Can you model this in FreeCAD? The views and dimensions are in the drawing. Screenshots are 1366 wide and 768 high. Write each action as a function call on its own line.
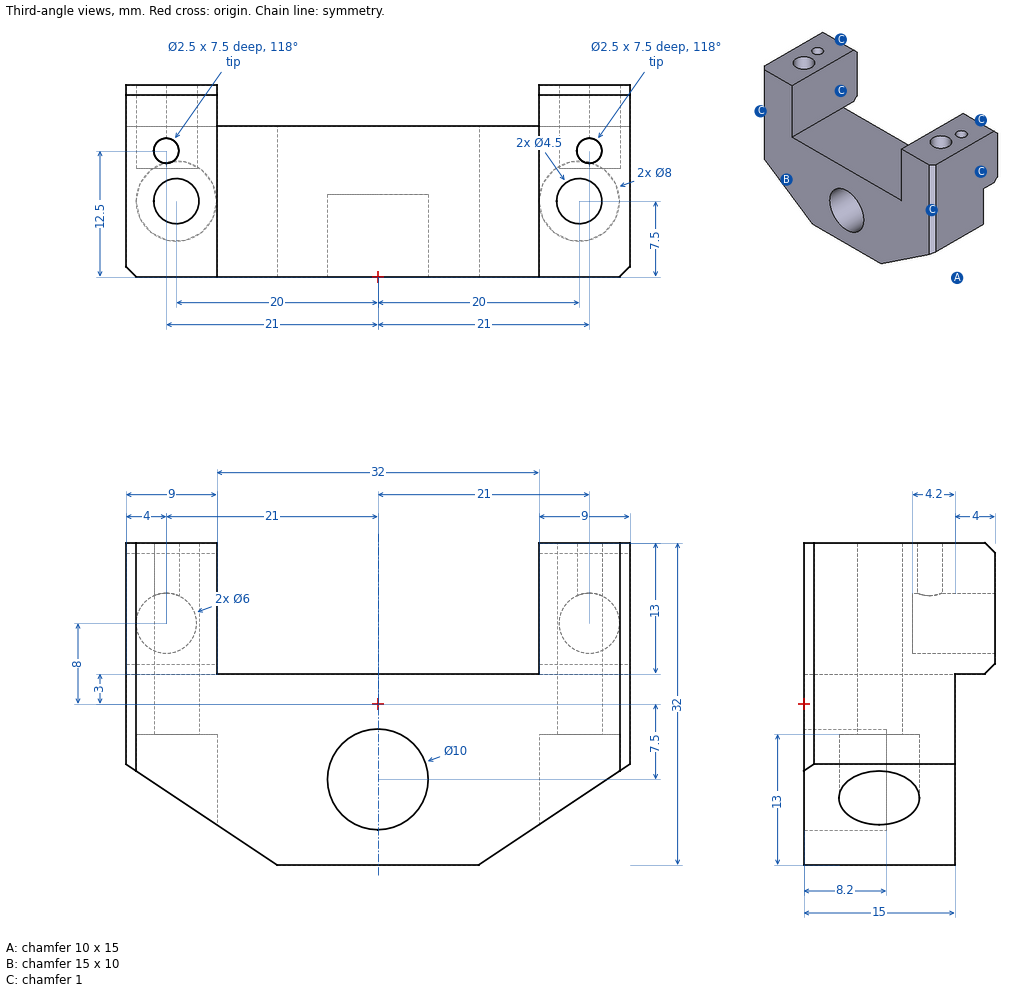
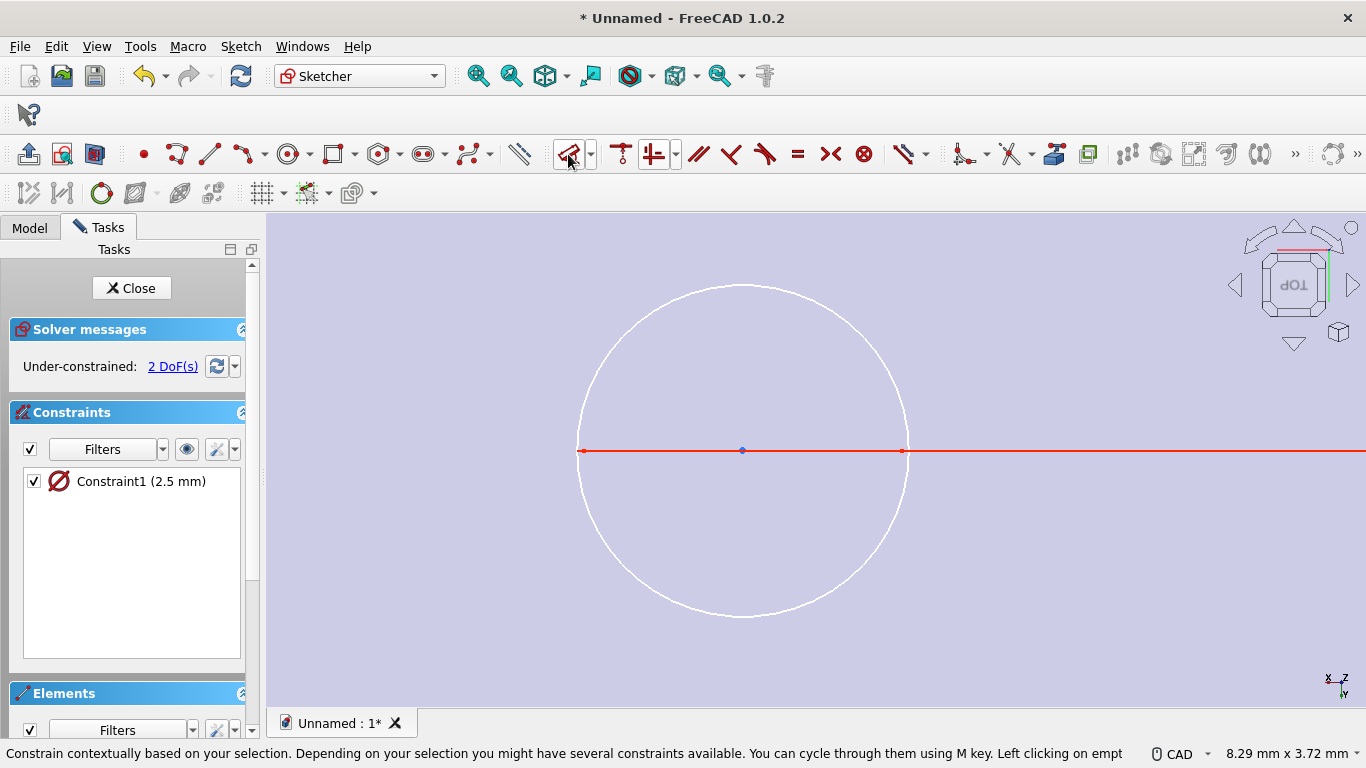
click(743, 451)
click(972, 485)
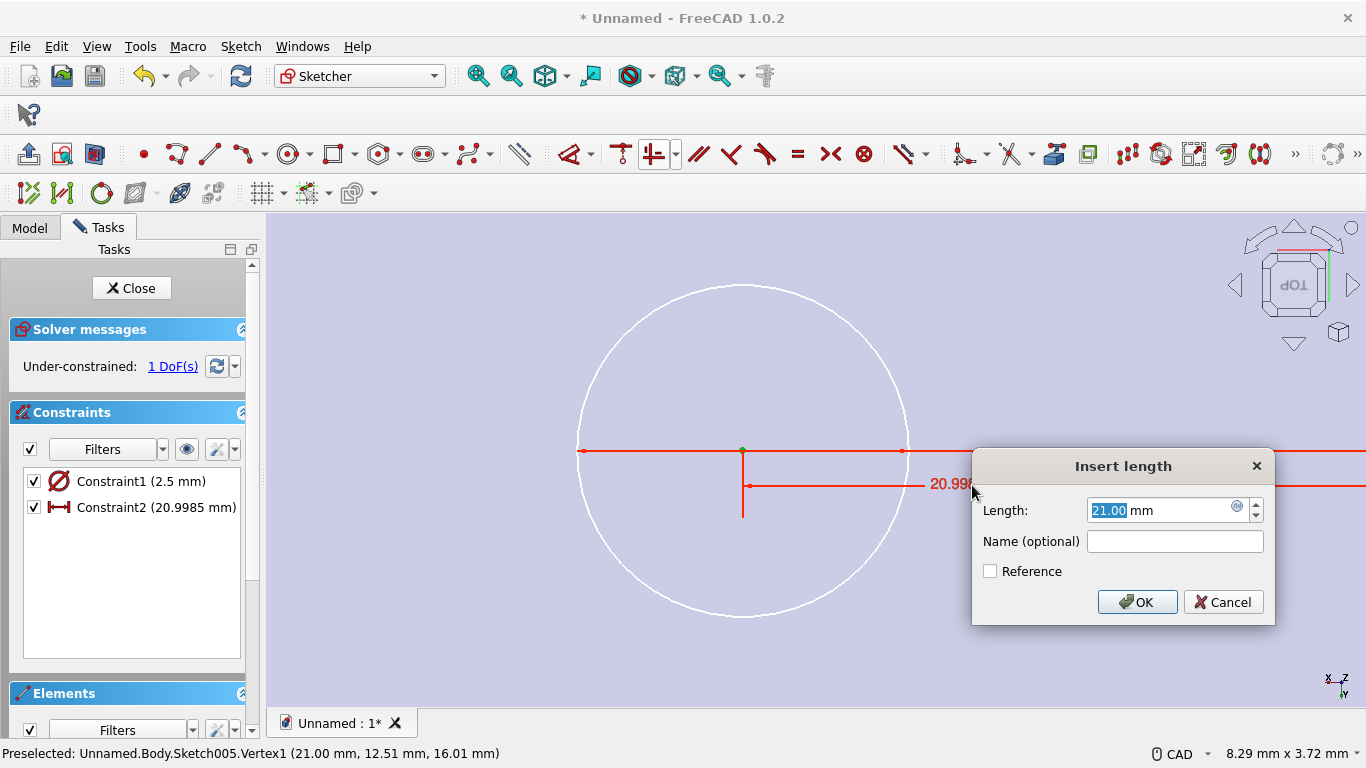
text(21)
key(Return)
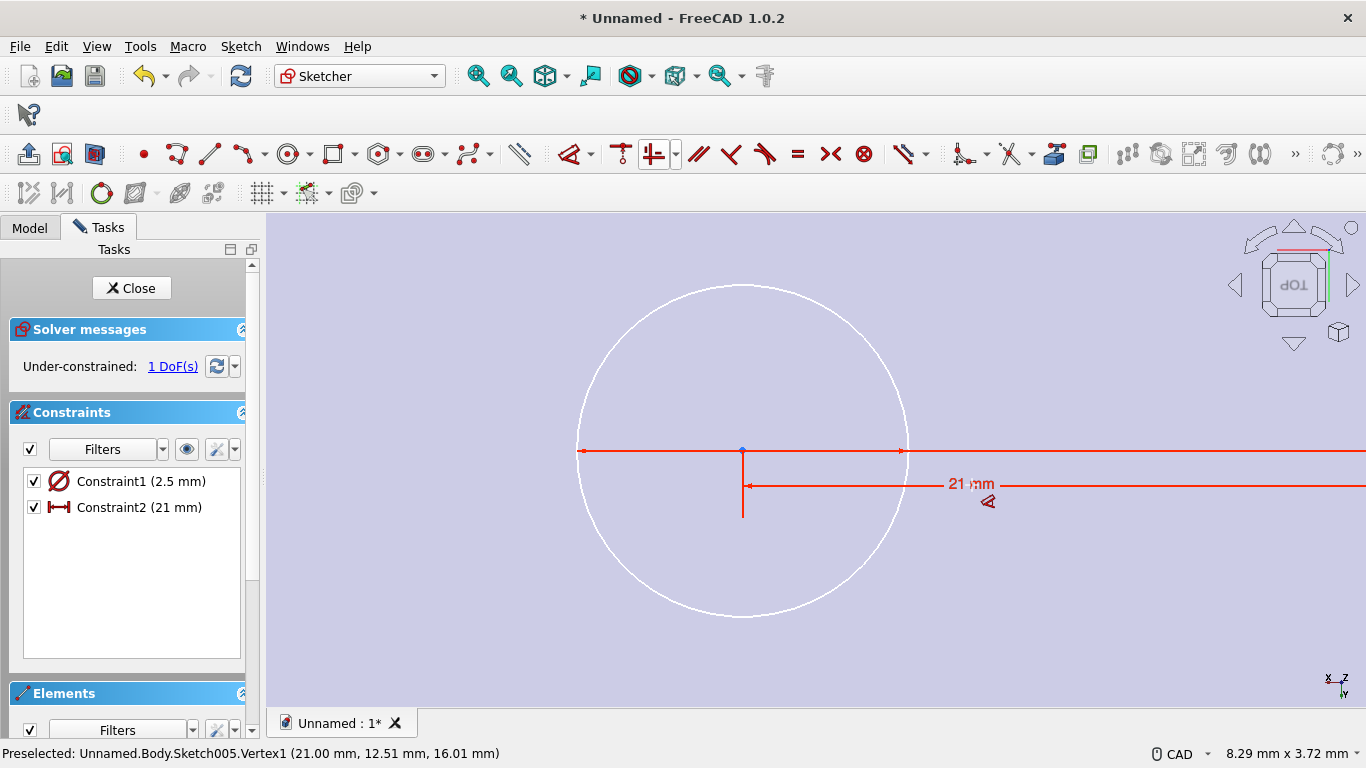
click(743, 451)
click(709, 346)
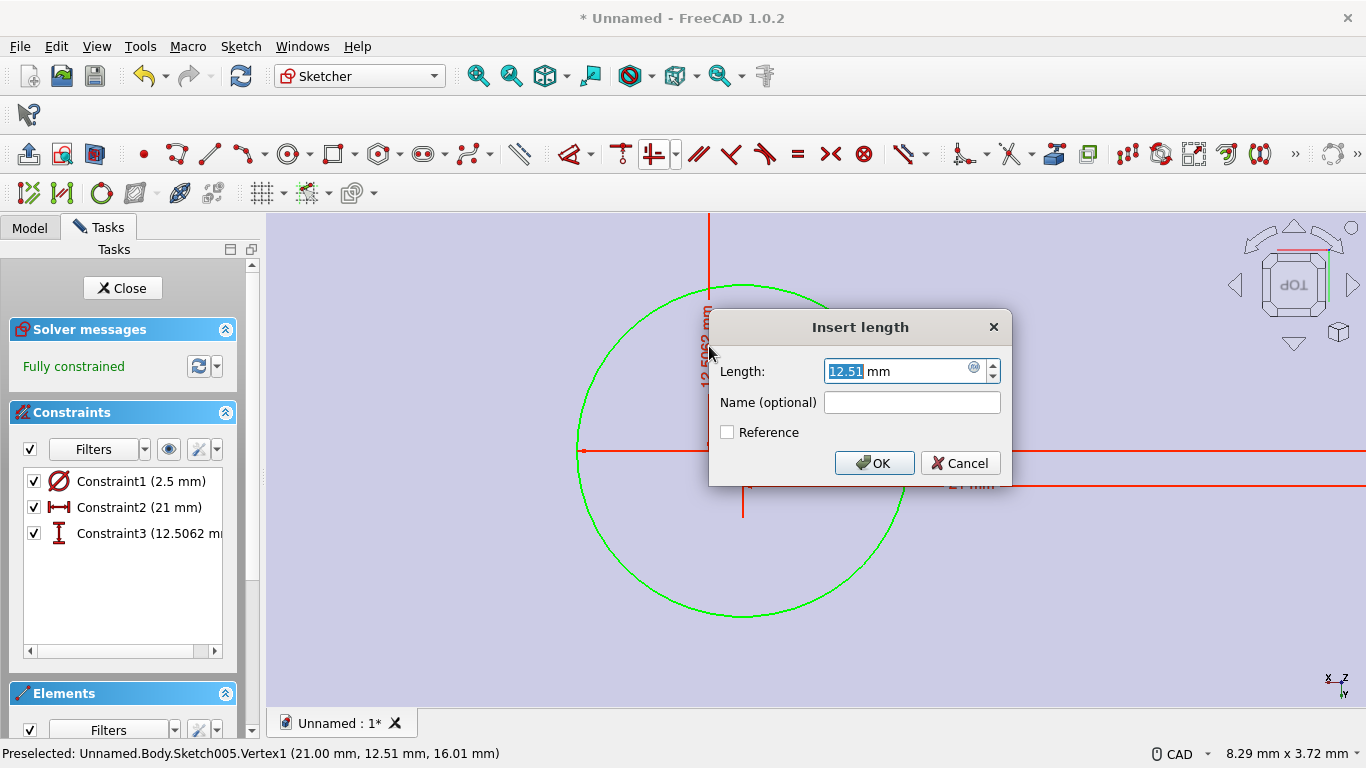
text(12.5)
key(Return)
key(Escape)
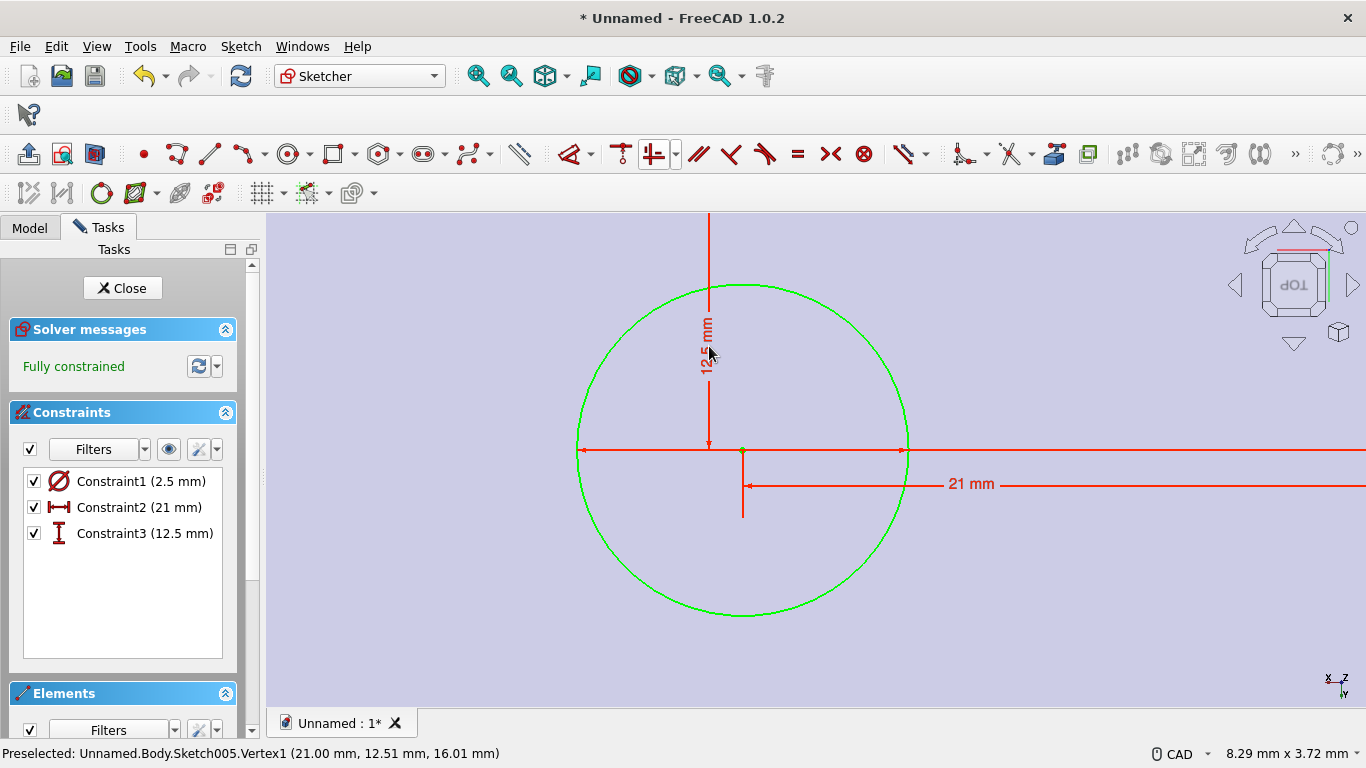
click(123, 288)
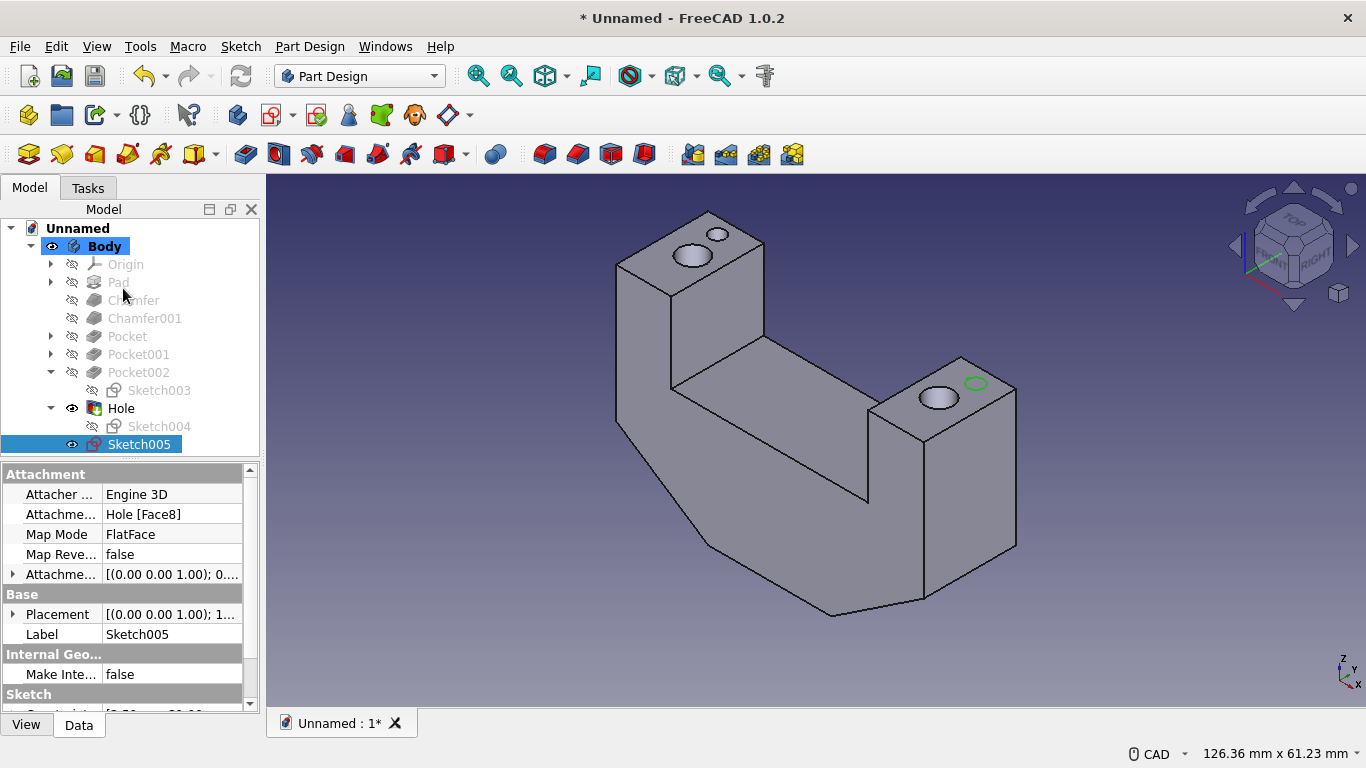
click(279, 154)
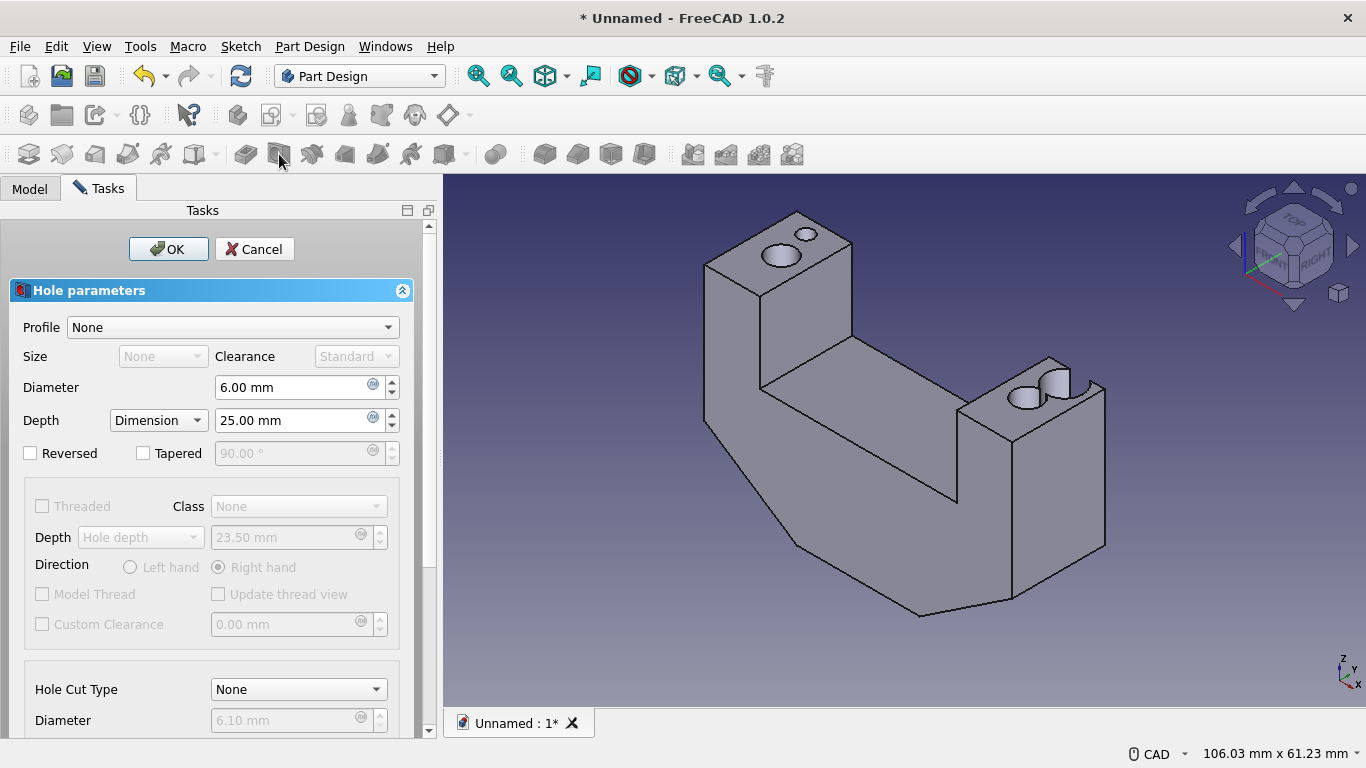
triple_click(300, 388)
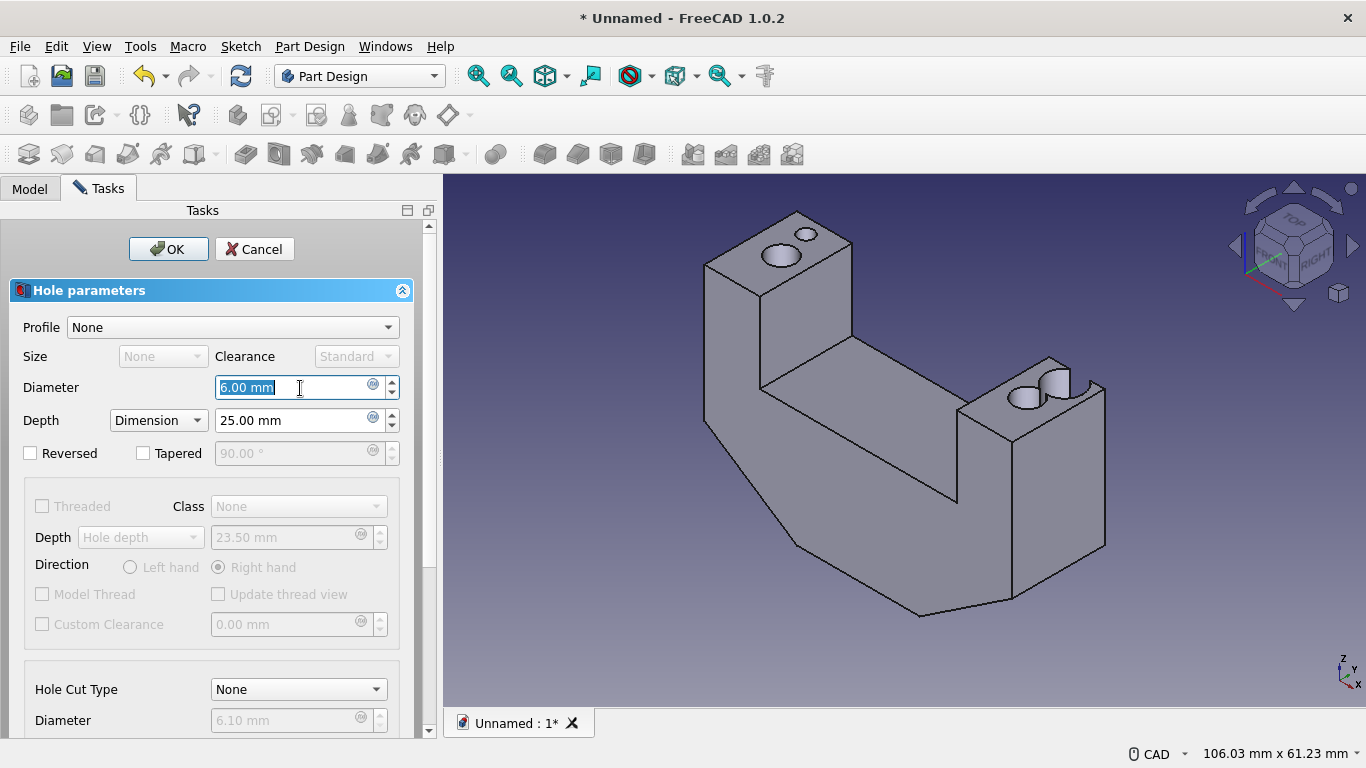
text(2.5)
key(Tab)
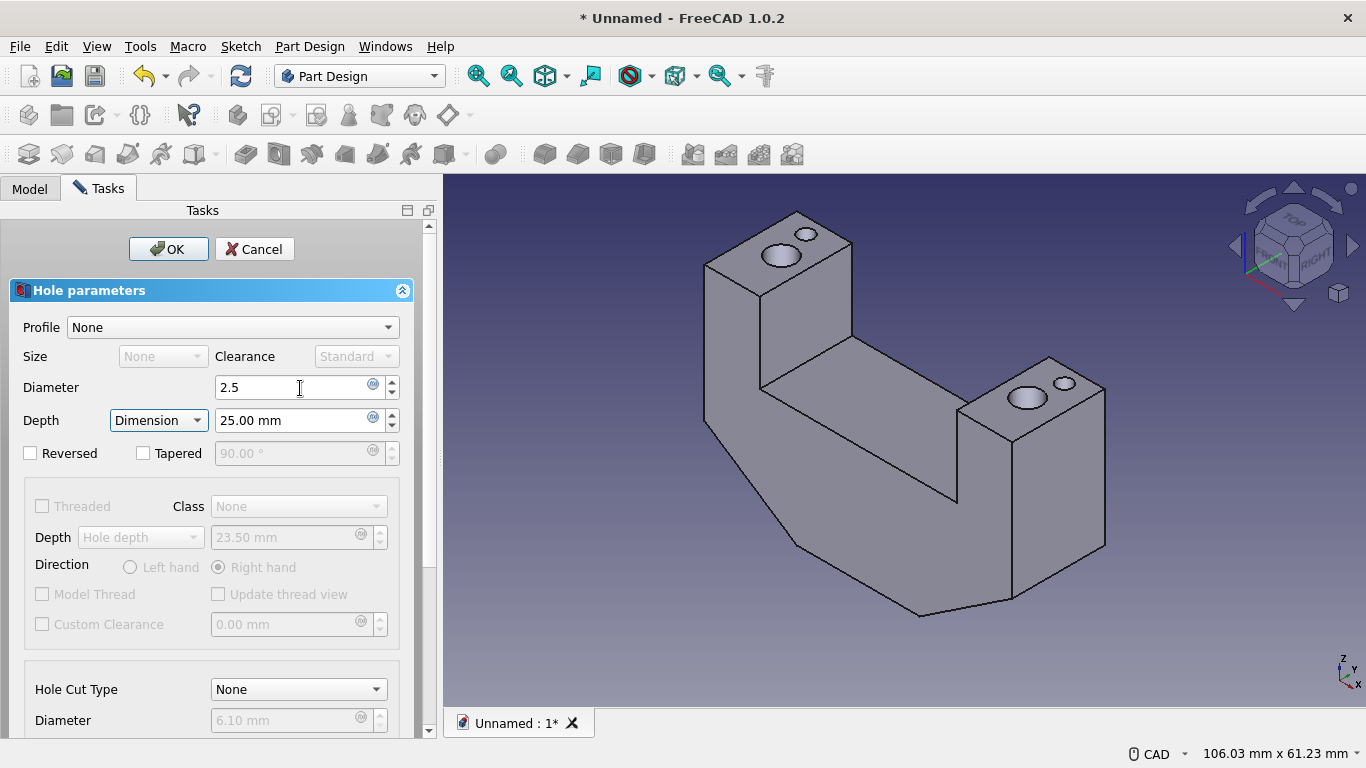
triple_click(300, 420)